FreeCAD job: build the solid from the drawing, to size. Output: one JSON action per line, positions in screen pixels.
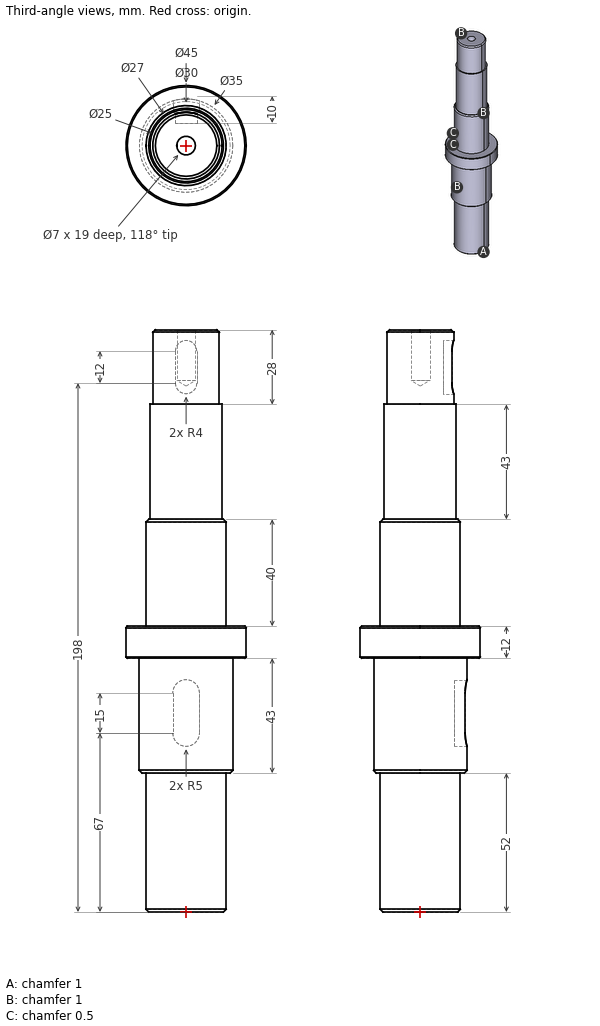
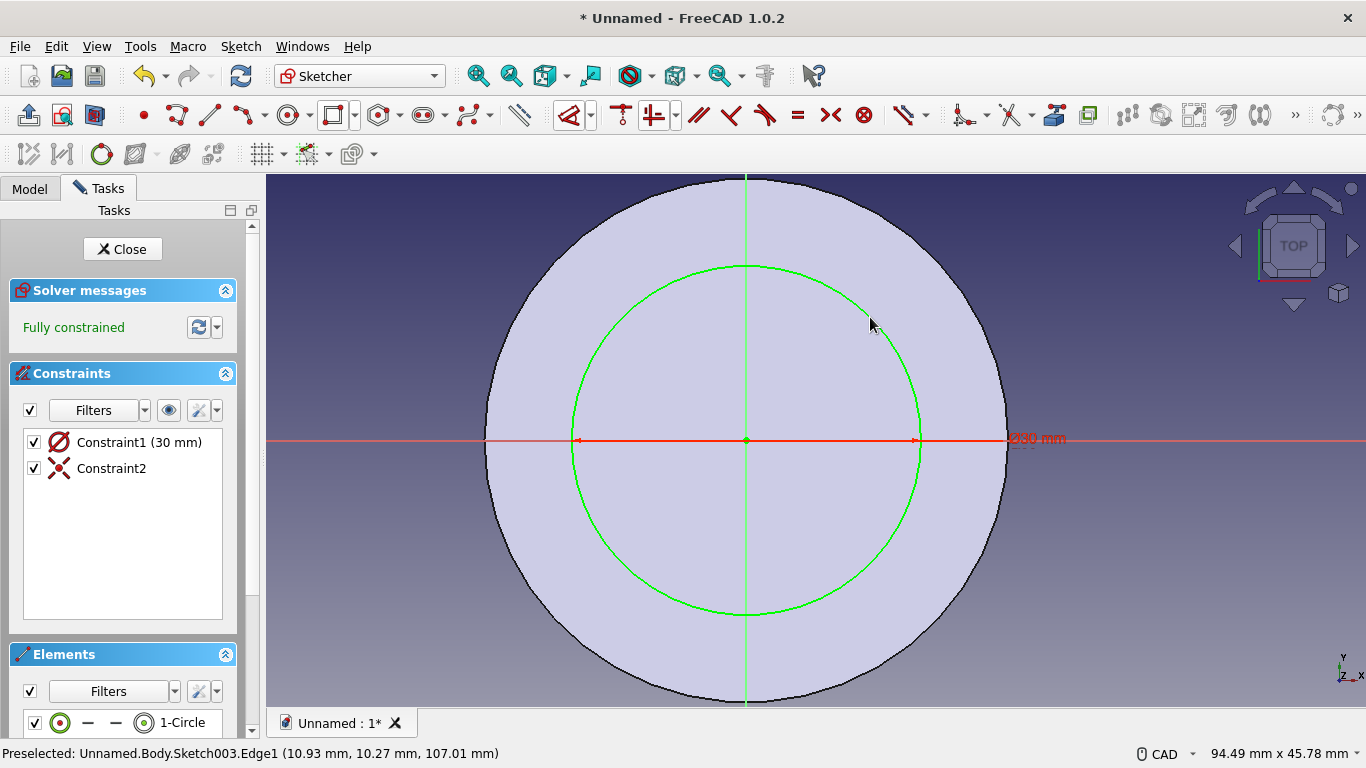
{"action": "left_click", "coordinate": [123, 249]}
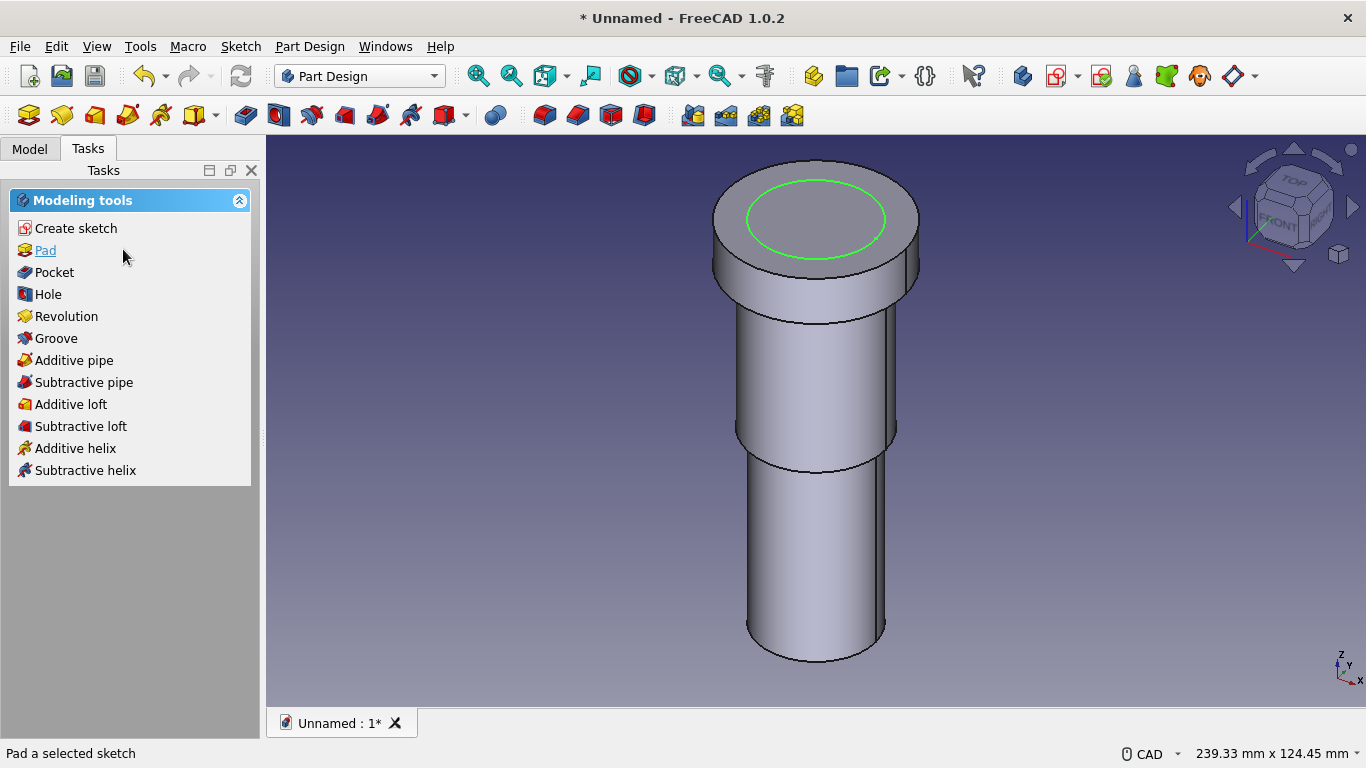
{"action": "left_click", "coordinate": [29, 116]}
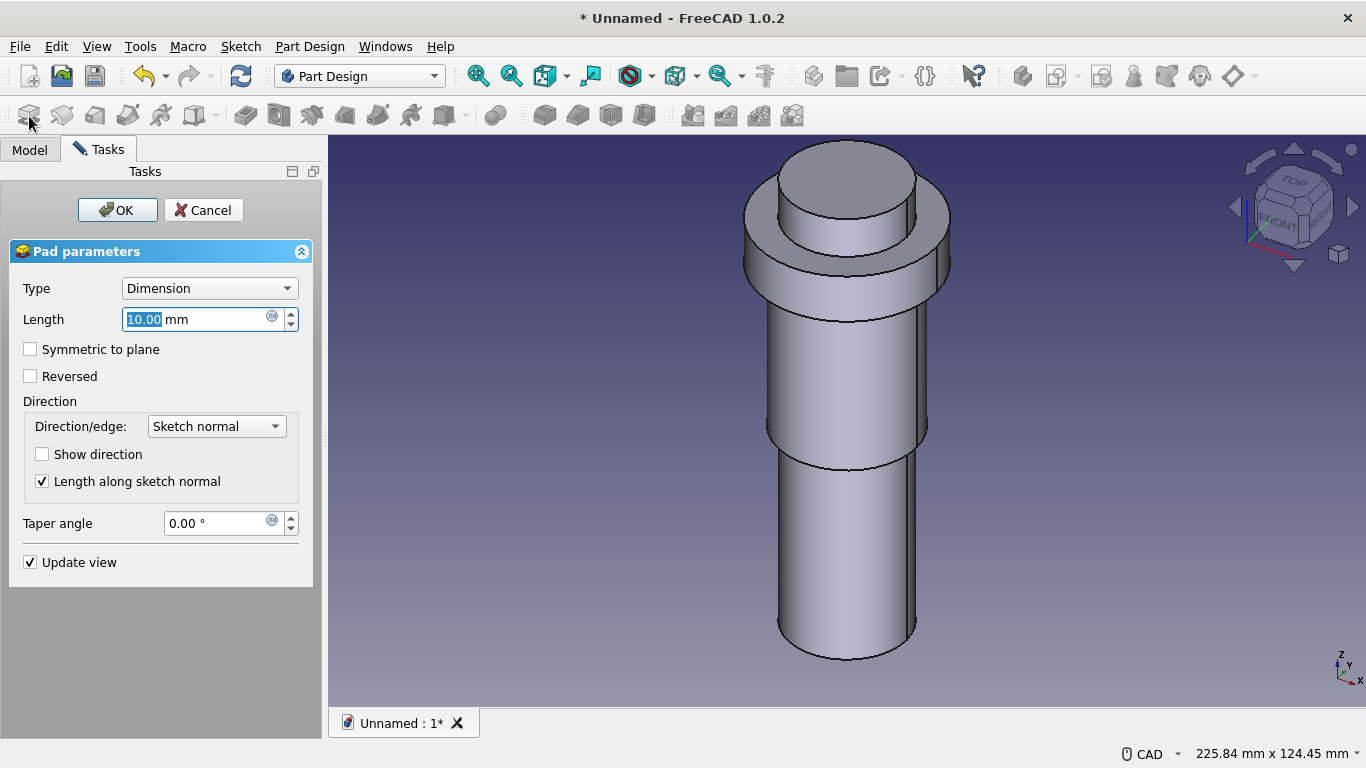
{"action": "type", "text": "40"}
{"action": "key", "text": "Tab"}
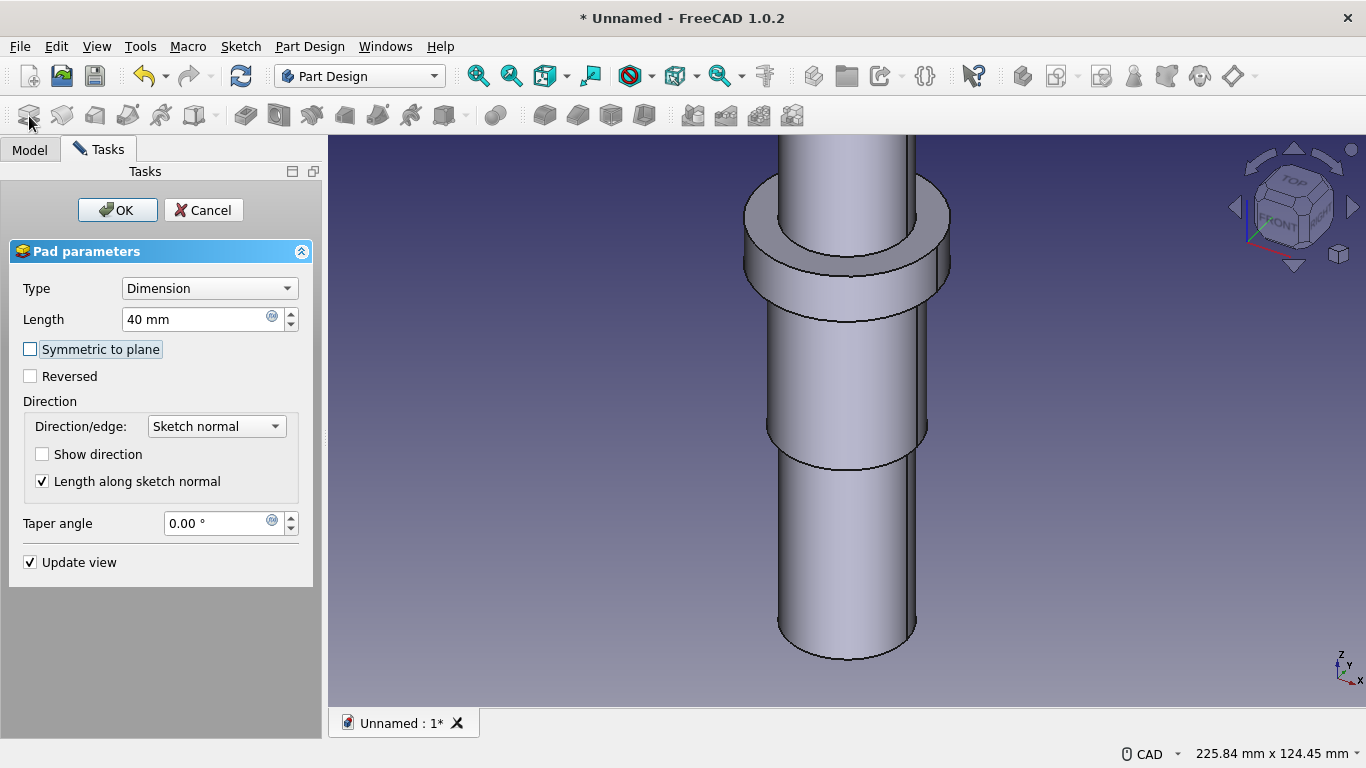
{"action": "left_click", "coordinate": [118, 210]}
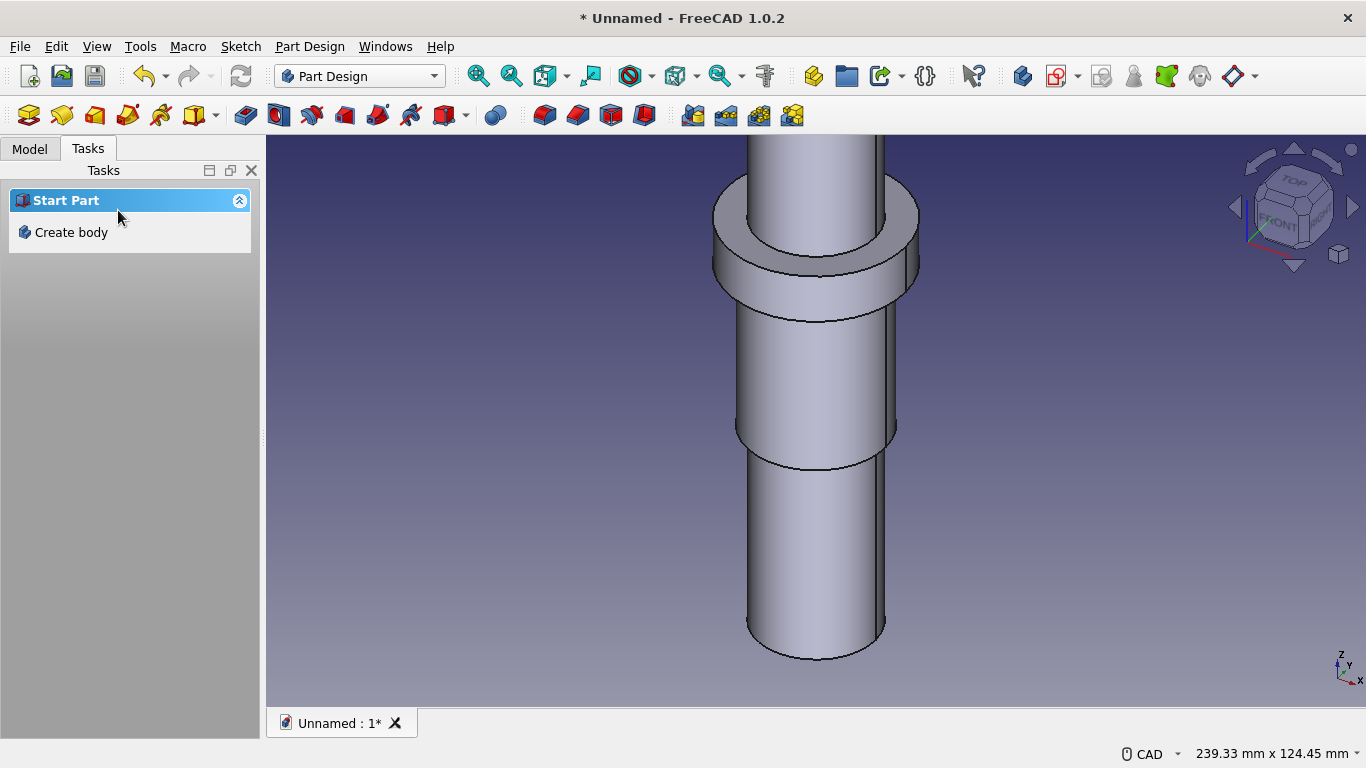
{"action": "key", "text": "v f"}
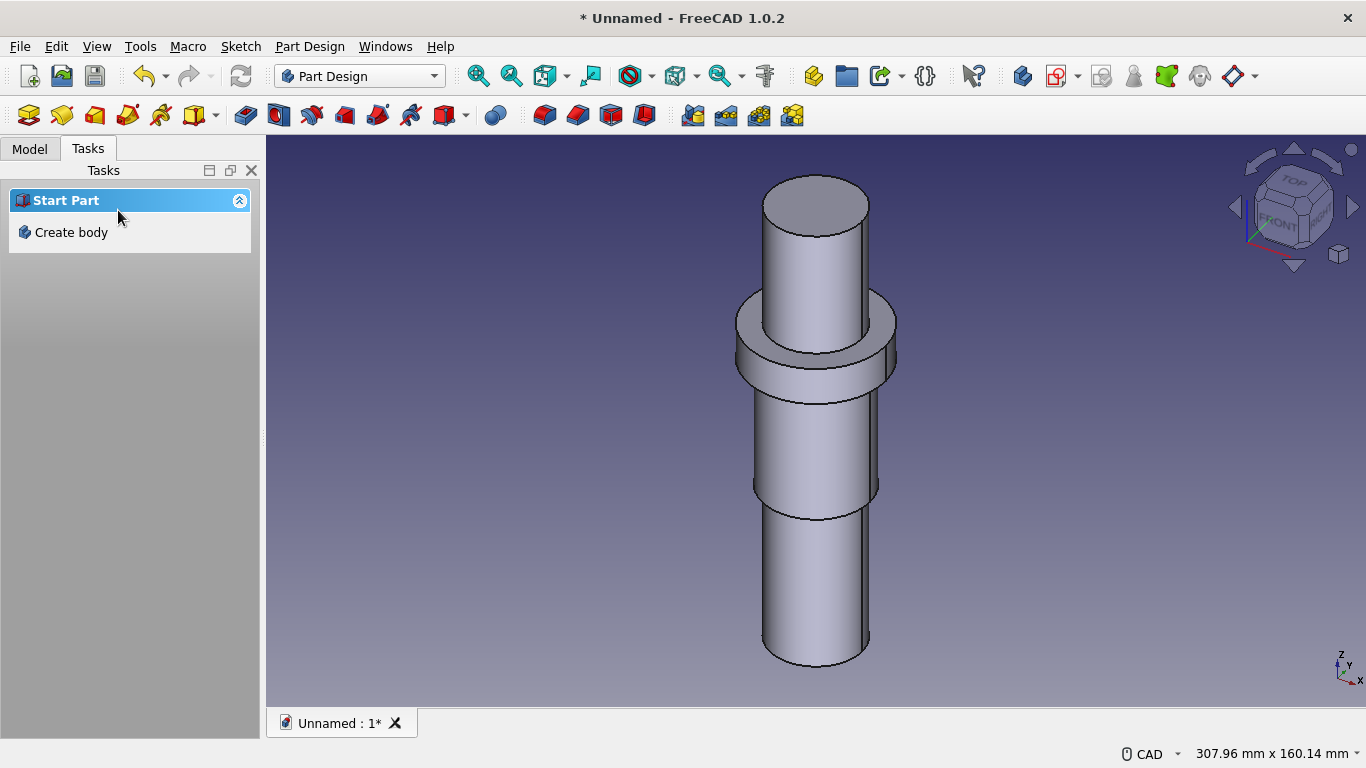
{"action": "left_click", "coordinate": [816, 205]}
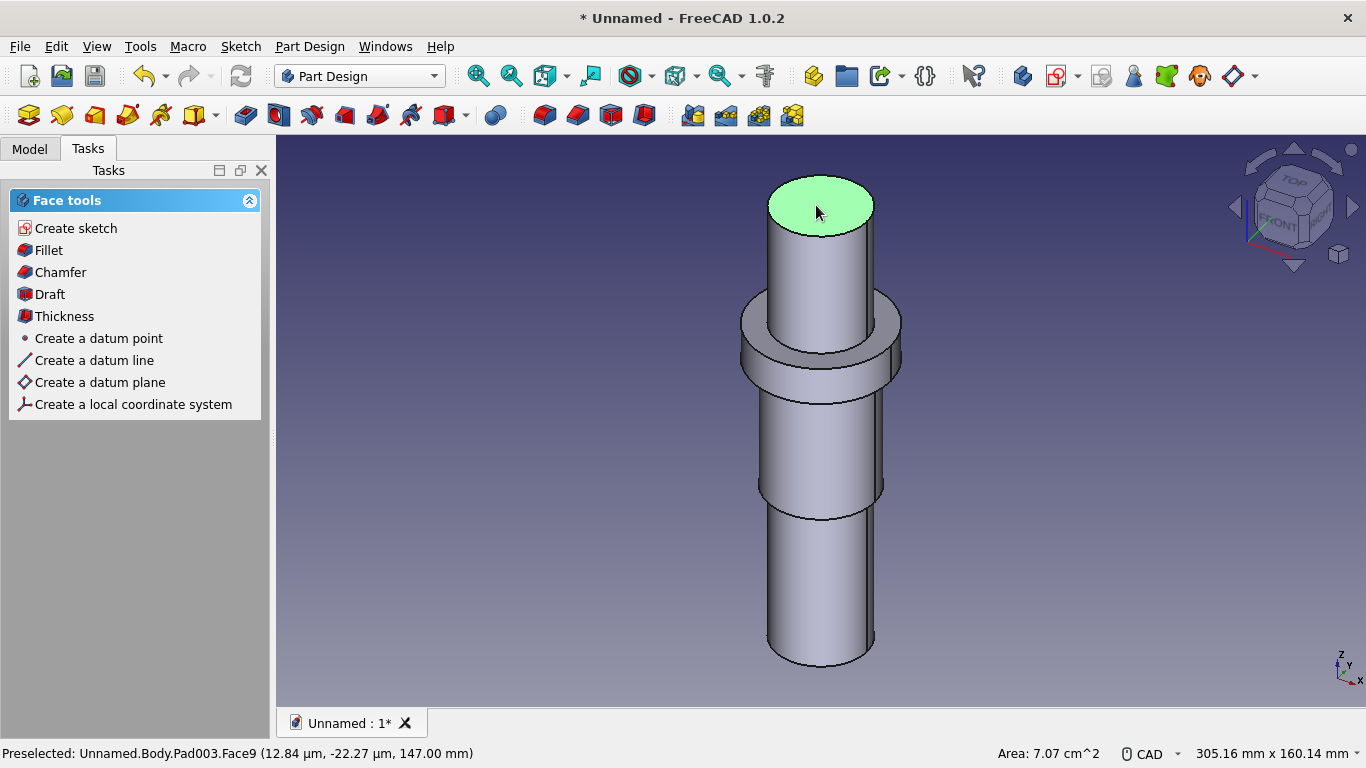
{"action": "left_click", "coordinate": [1056, 76]}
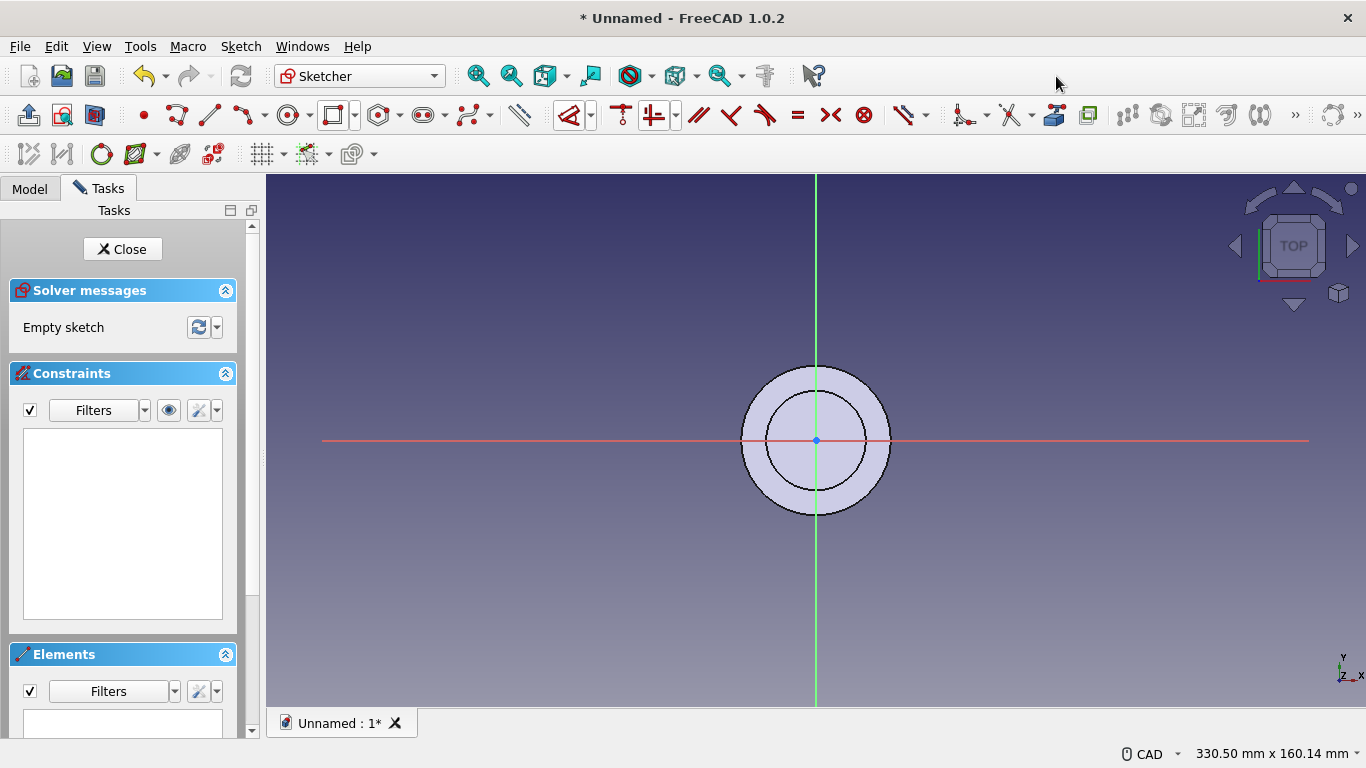
{"action": "scroll", "coordinate": [838, 440], "scroll_direction": "up", "scroll_amount": 7}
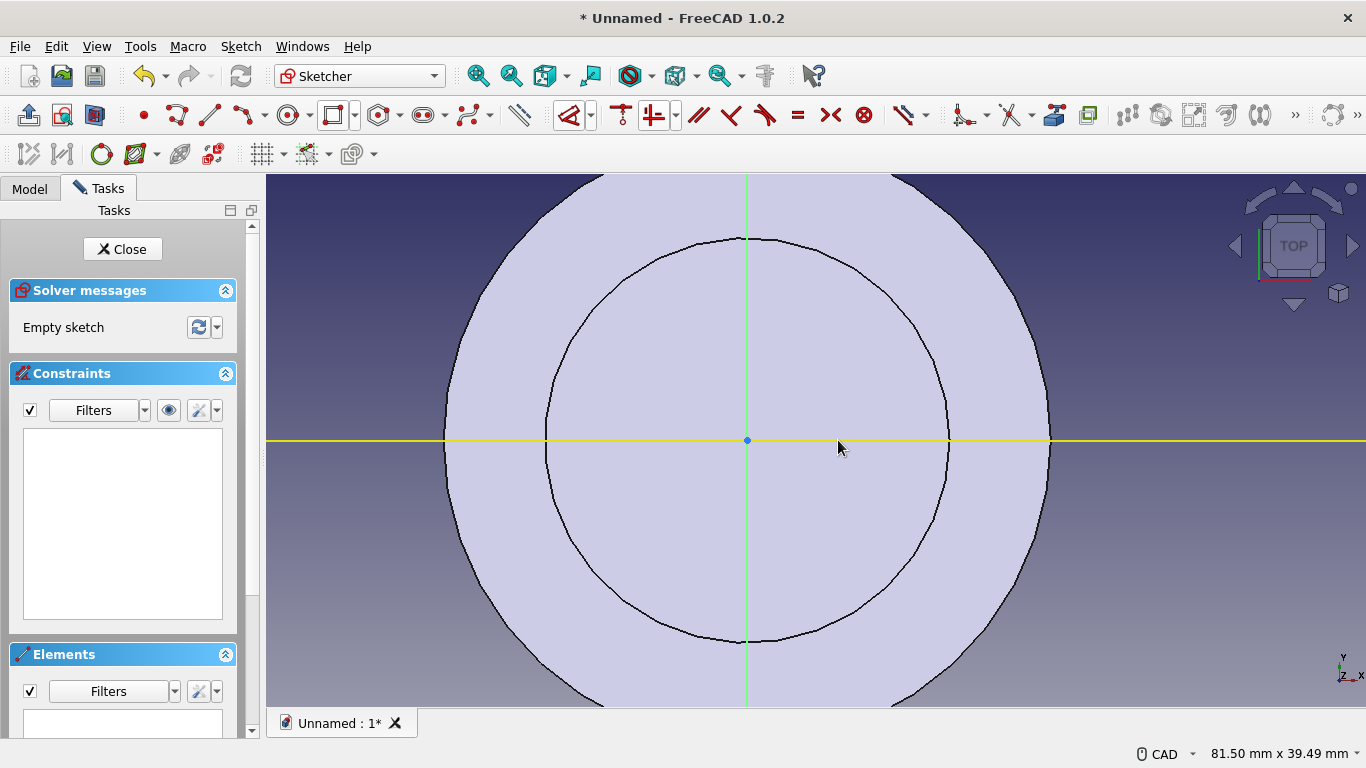
{"action": "key", "text": "g c"}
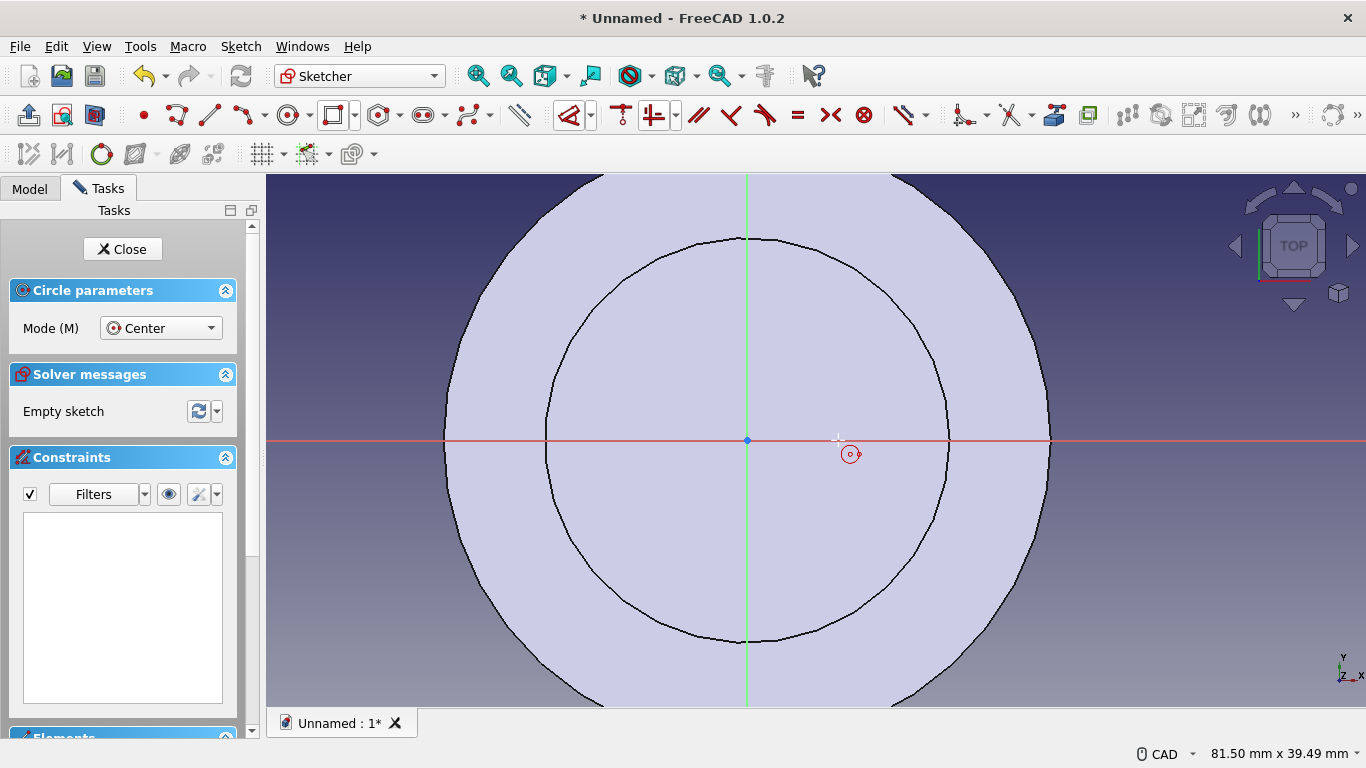
{"action": "left_click", "coordinate": [747, 440]}
{"action": "mouse_move", "coordinate": [876, 312]}